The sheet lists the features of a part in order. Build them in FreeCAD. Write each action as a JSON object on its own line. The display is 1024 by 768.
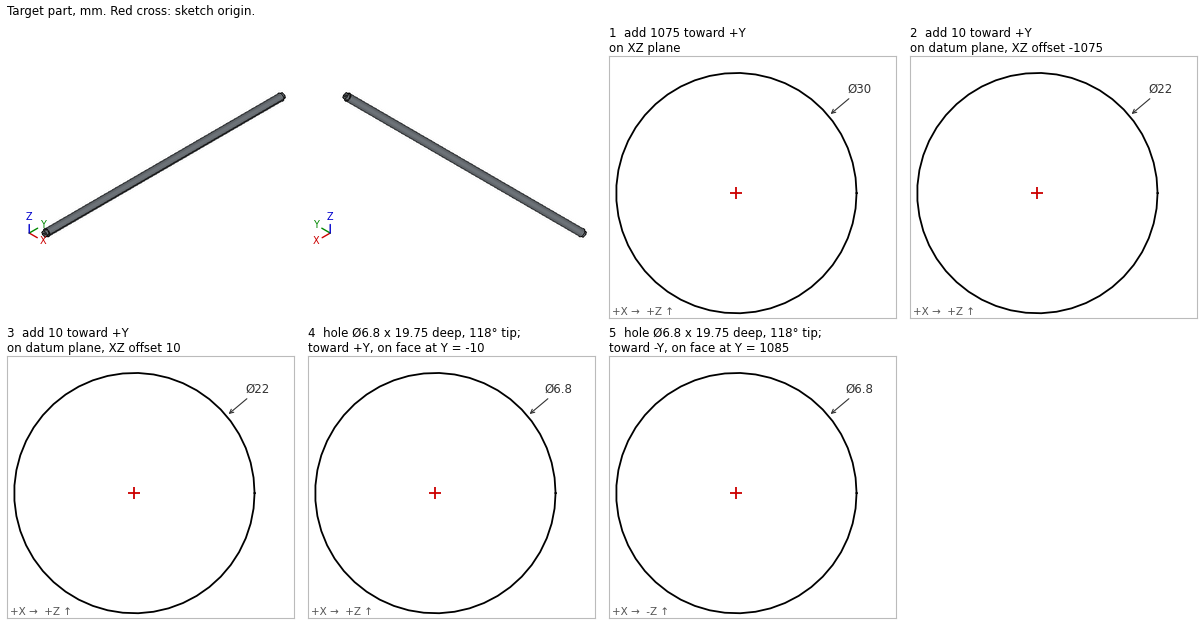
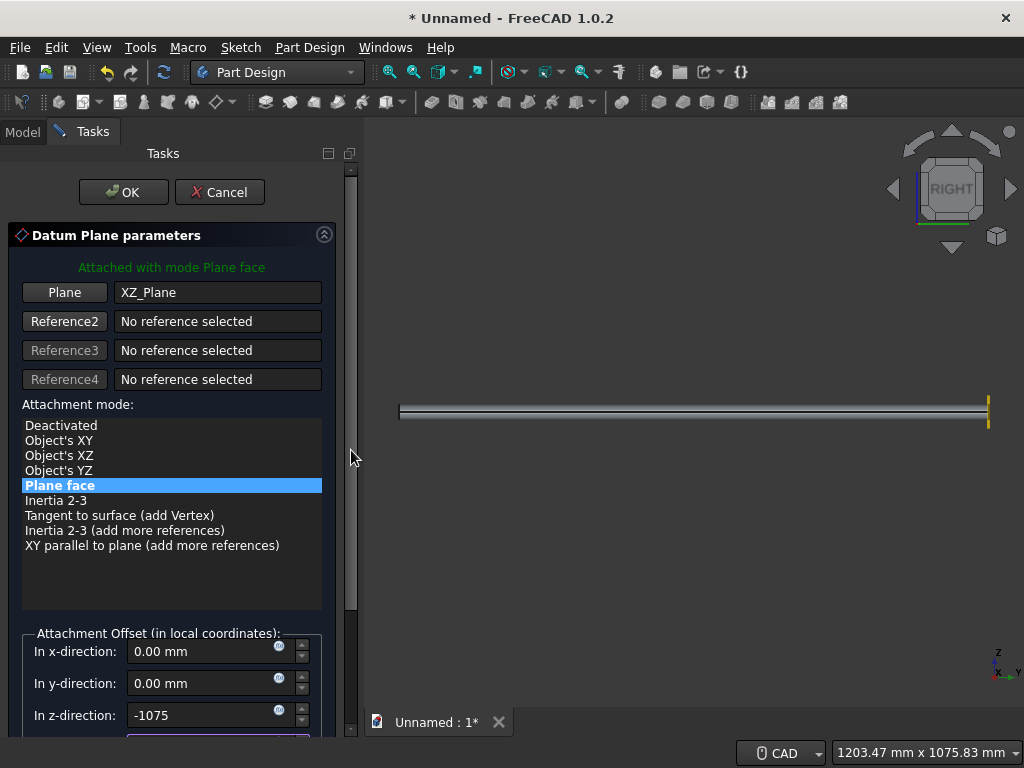
{"action": "left_click", "coordinate": [124, 192]}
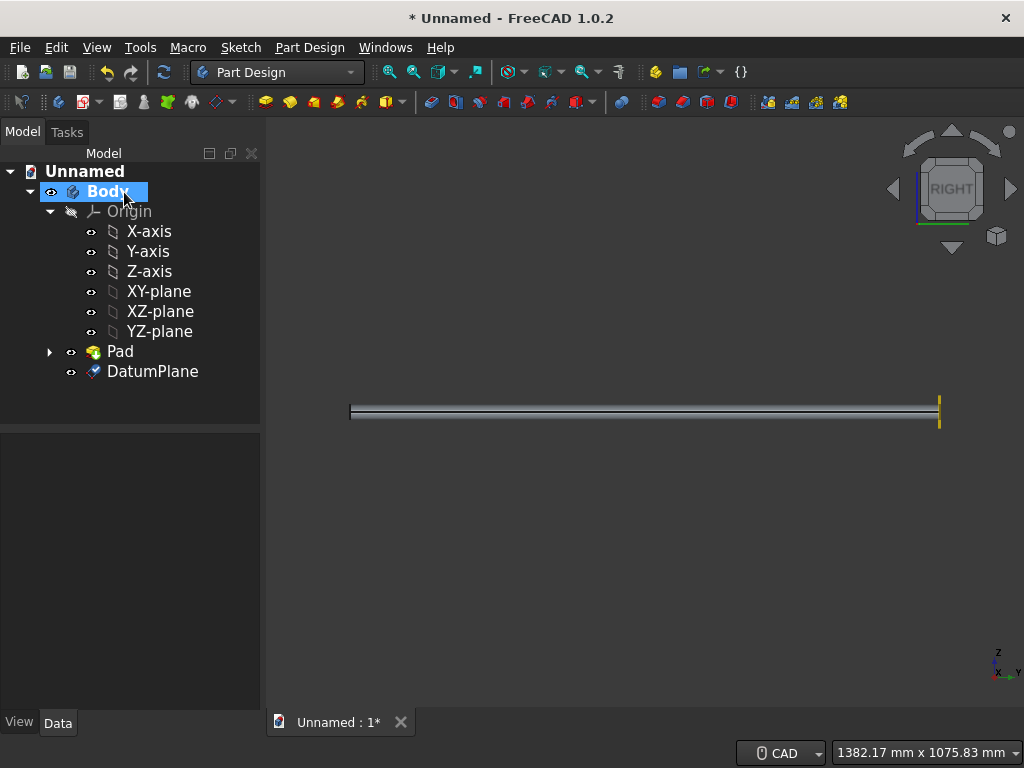
{"action": "left_click", "coordinate": [116, 372]}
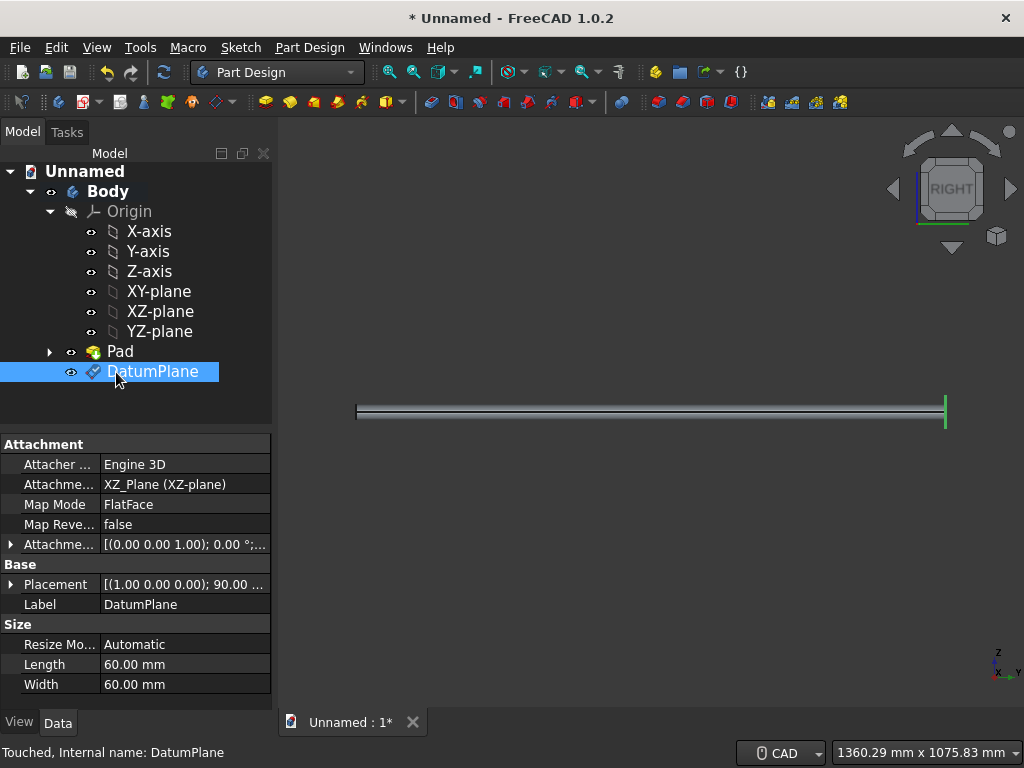
{"action": "left_click", "coordinate": [84, 102]}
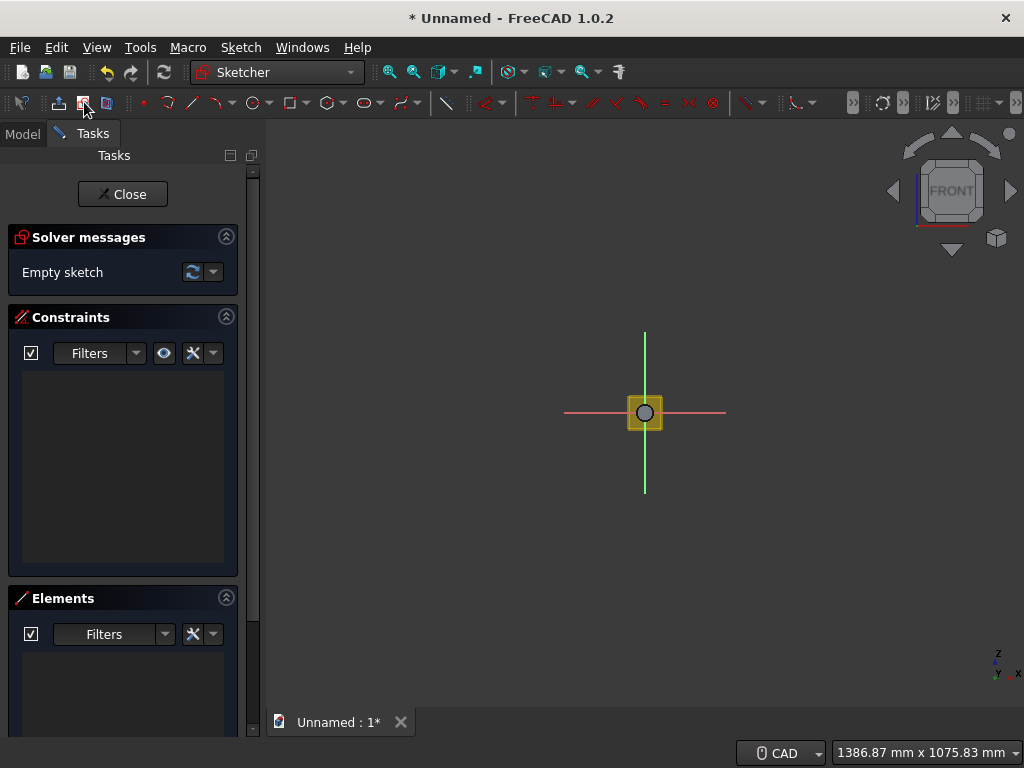
{"action": "left_click", "coordinate": [108, 104]}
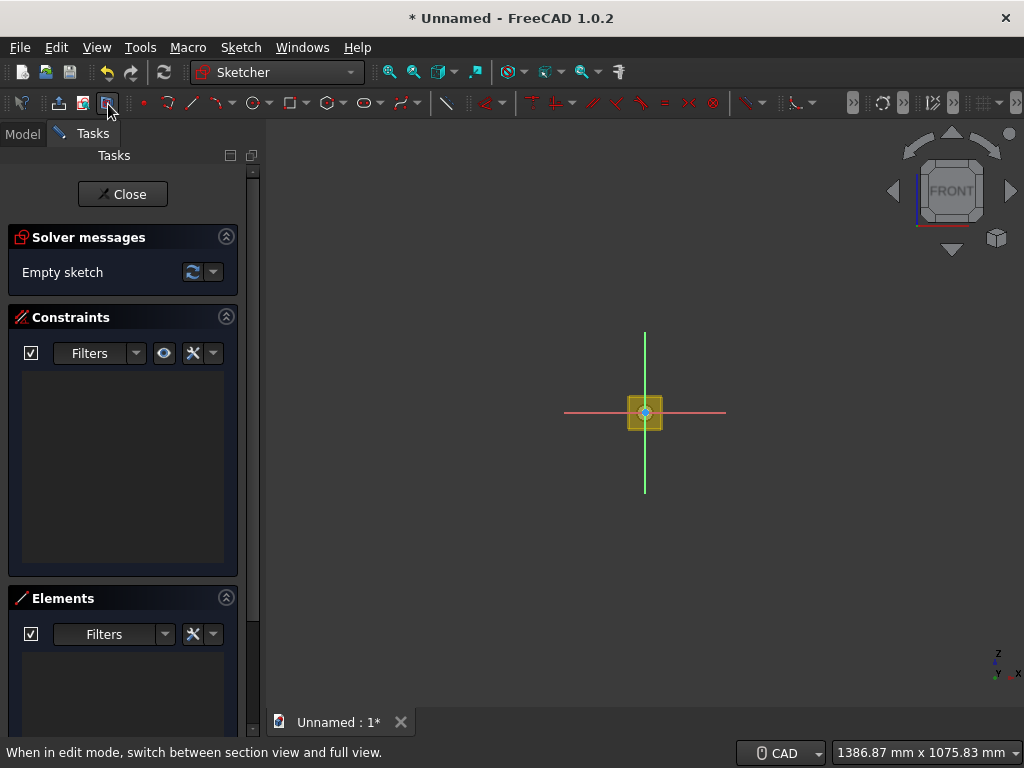
{"action": "scroll", "coordinate": [649, 413], "scroll_direction": "up", "scroll_amount": 15}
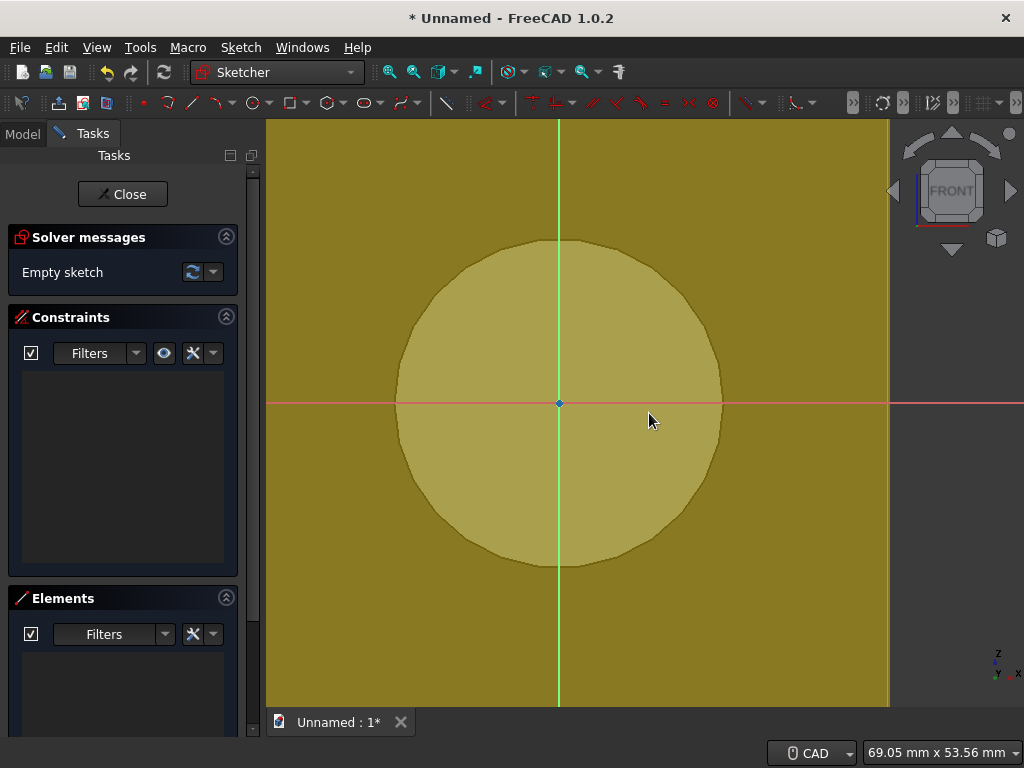
{"action": "scroll", "coordinate": [523, 384], "scroll_direction": "up", "scroll_amount": 2}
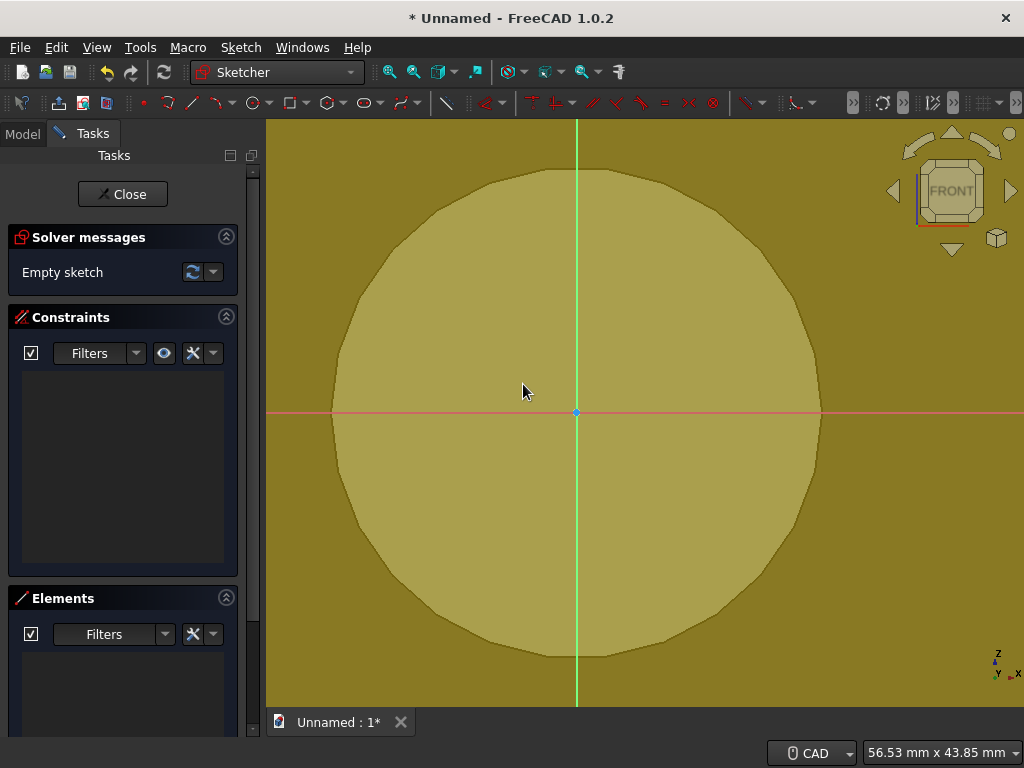
{"action": "left_click", "coordinate": [254, 104]}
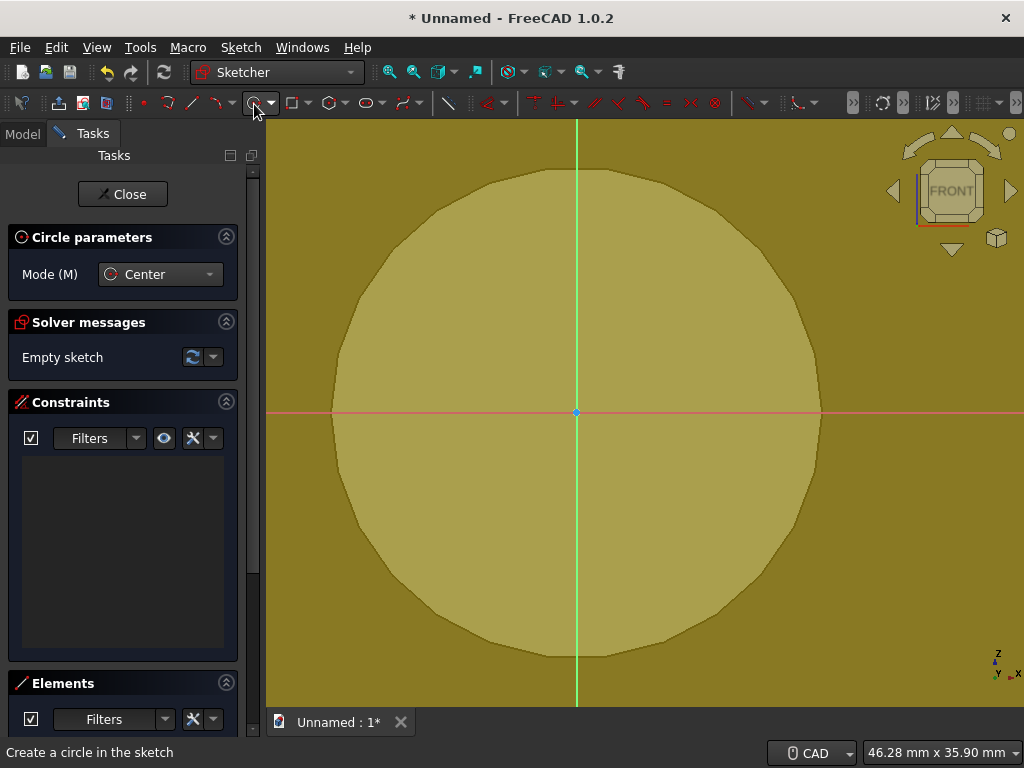
{"action": "left_click", "coordinate": [577, 413]}
{"action": "mouse_move", "coordinate": [704, 285]}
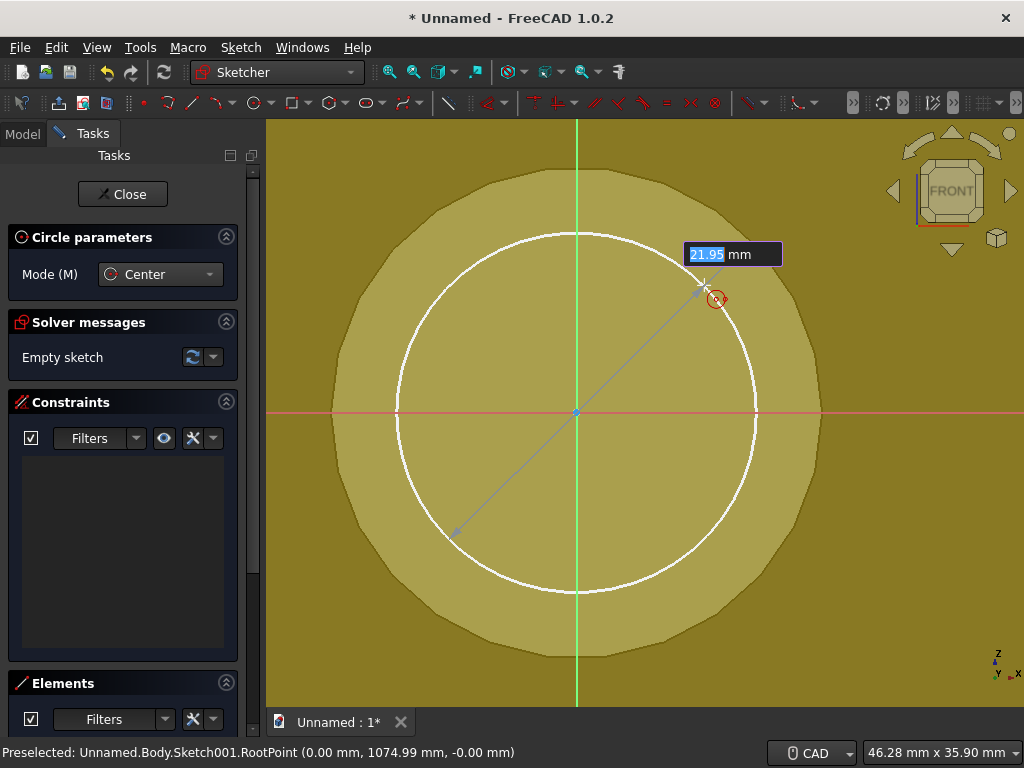
{"action": "type", "text": "22"}
{"action": "key", "text": "Return"}
{"action": "key", "text": "Escape"}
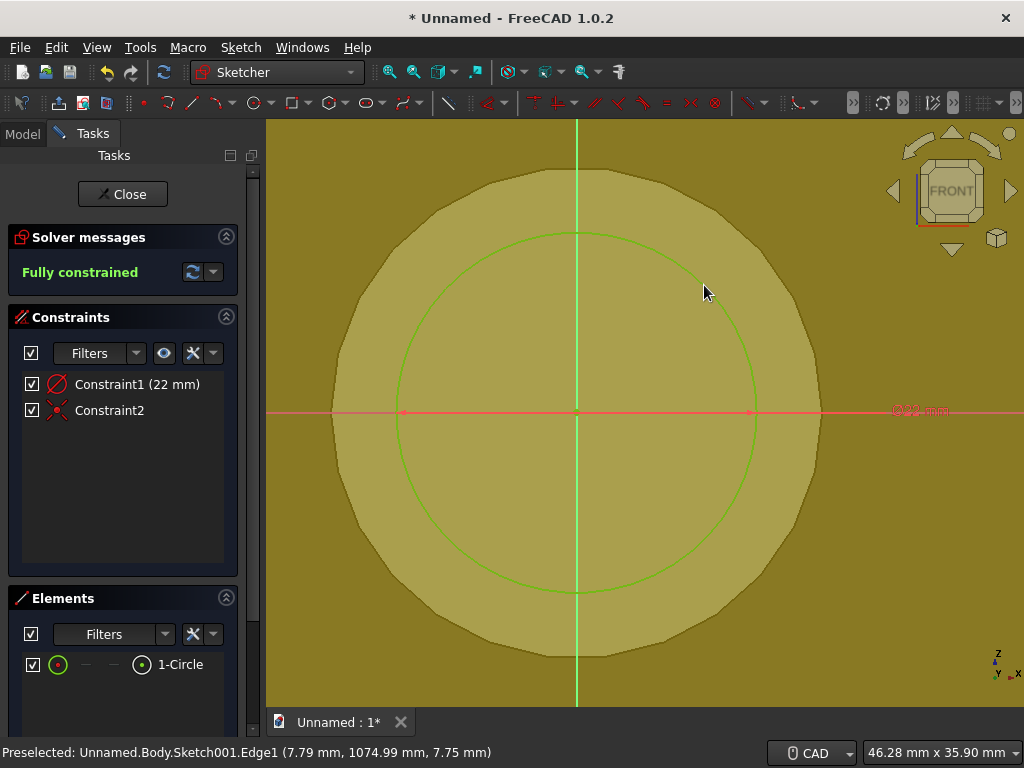
{"action": "left_click", "coordinate": [123, 194]}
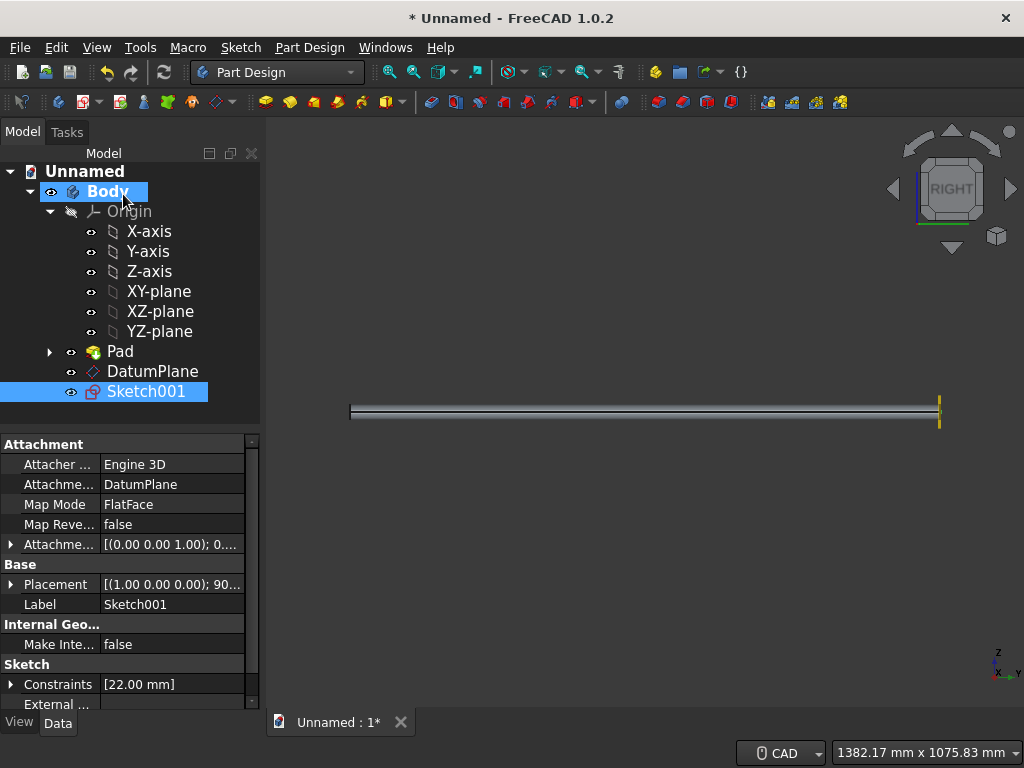
{"action": "left_click", "coordinate": [266, 102]}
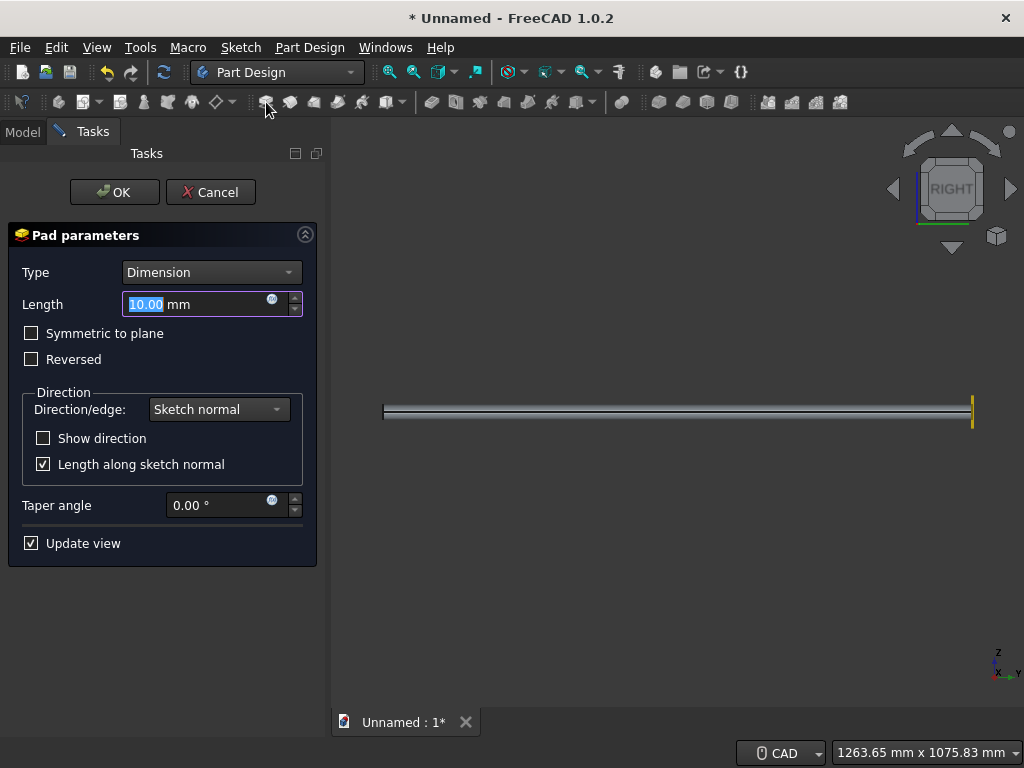
{"action": "type", "text": "10"}
{"action": "key", "text": "Tab"}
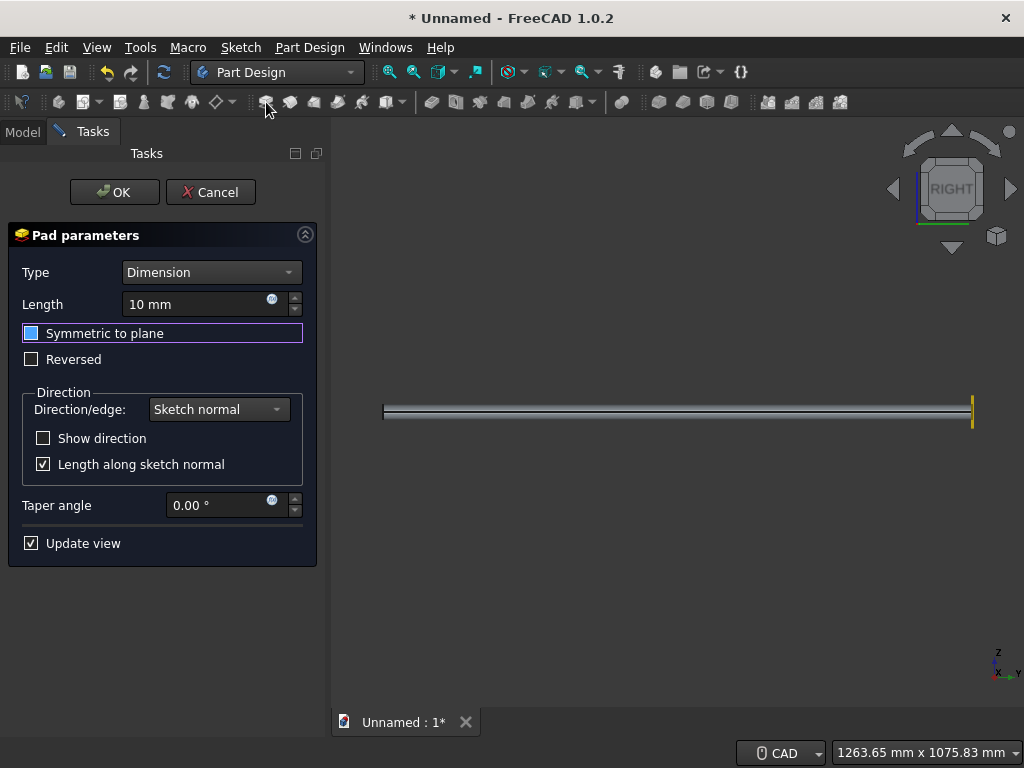
{"action": "left_click", "coordinate": [30, 359]}